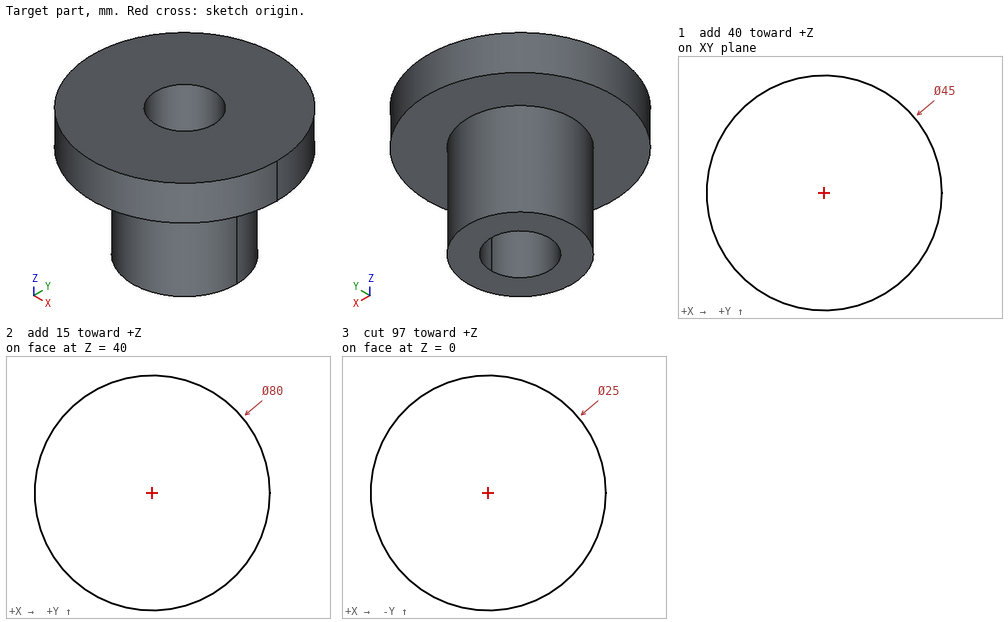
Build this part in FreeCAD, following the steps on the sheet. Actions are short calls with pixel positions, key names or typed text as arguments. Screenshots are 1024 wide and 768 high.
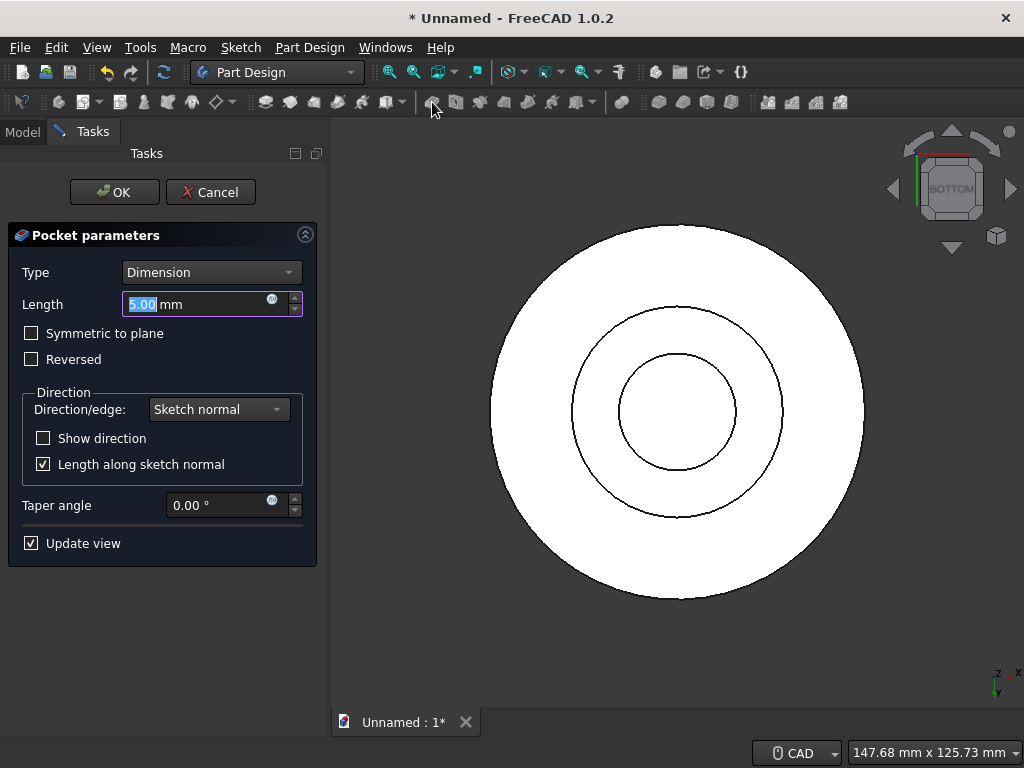
text(97)
key(Tab)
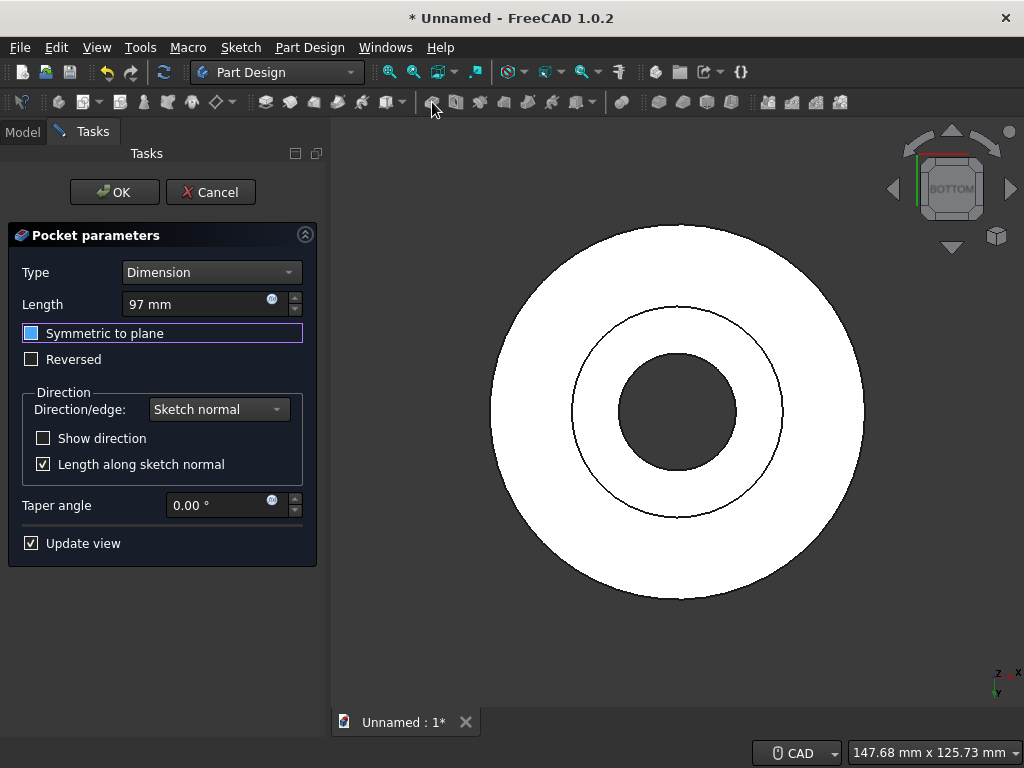
click(115, 192)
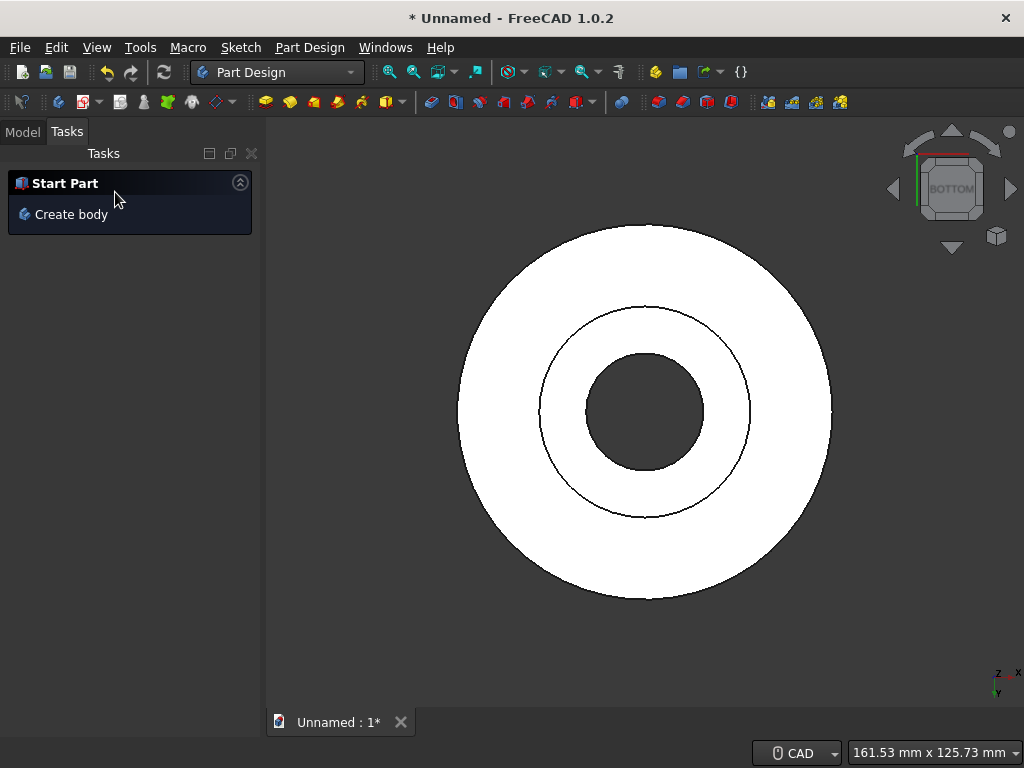
key(0)